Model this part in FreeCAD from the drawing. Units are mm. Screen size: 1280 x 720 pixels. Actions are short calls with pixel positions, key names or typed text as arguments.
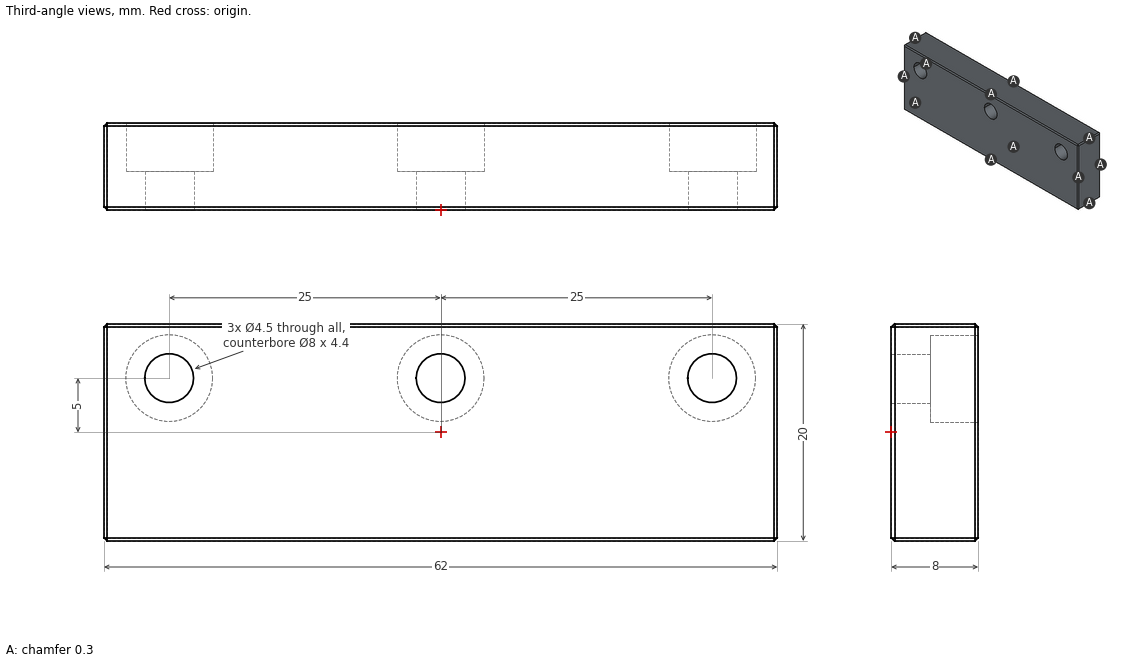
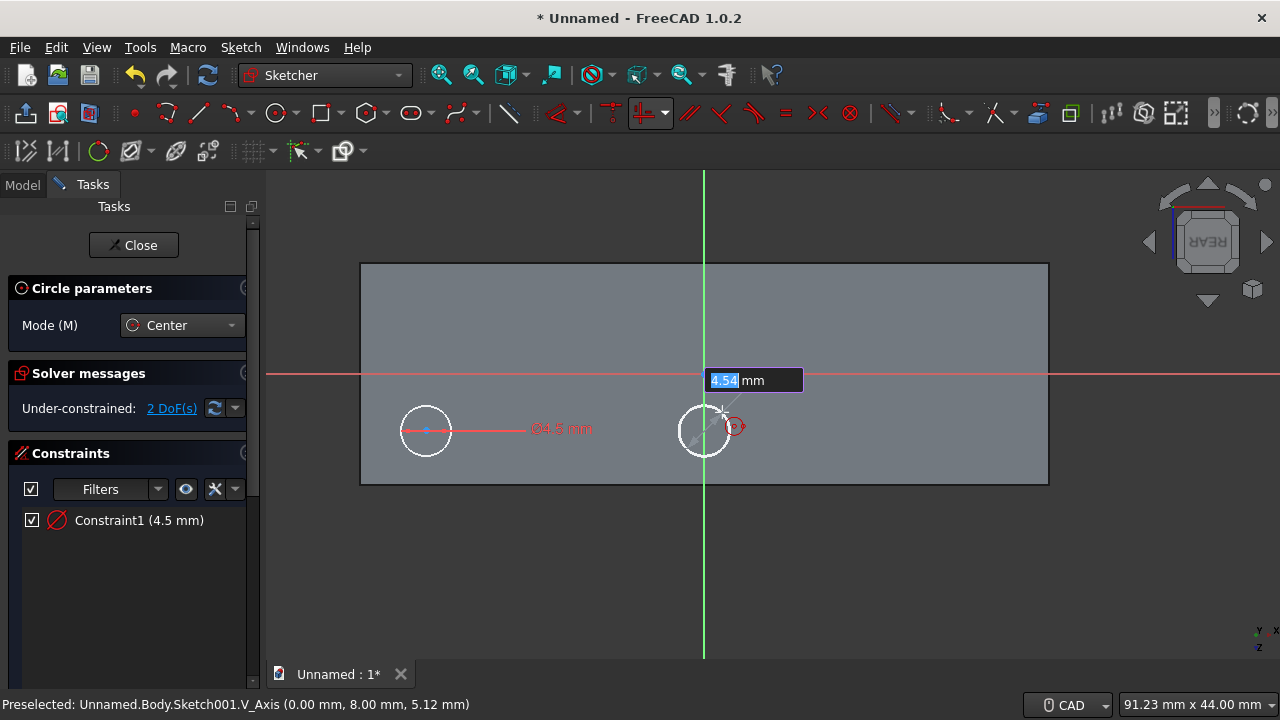
text(4.5)
key(Return)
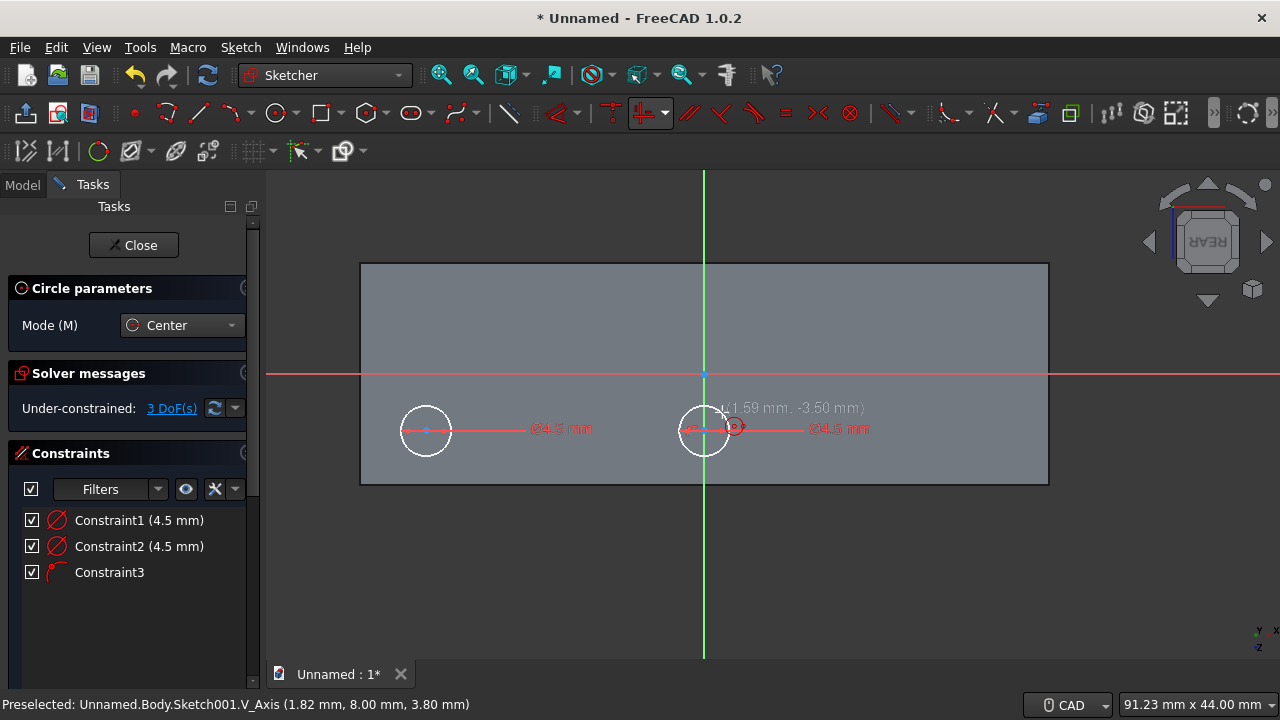
click(982, 430)
move(1000, 412)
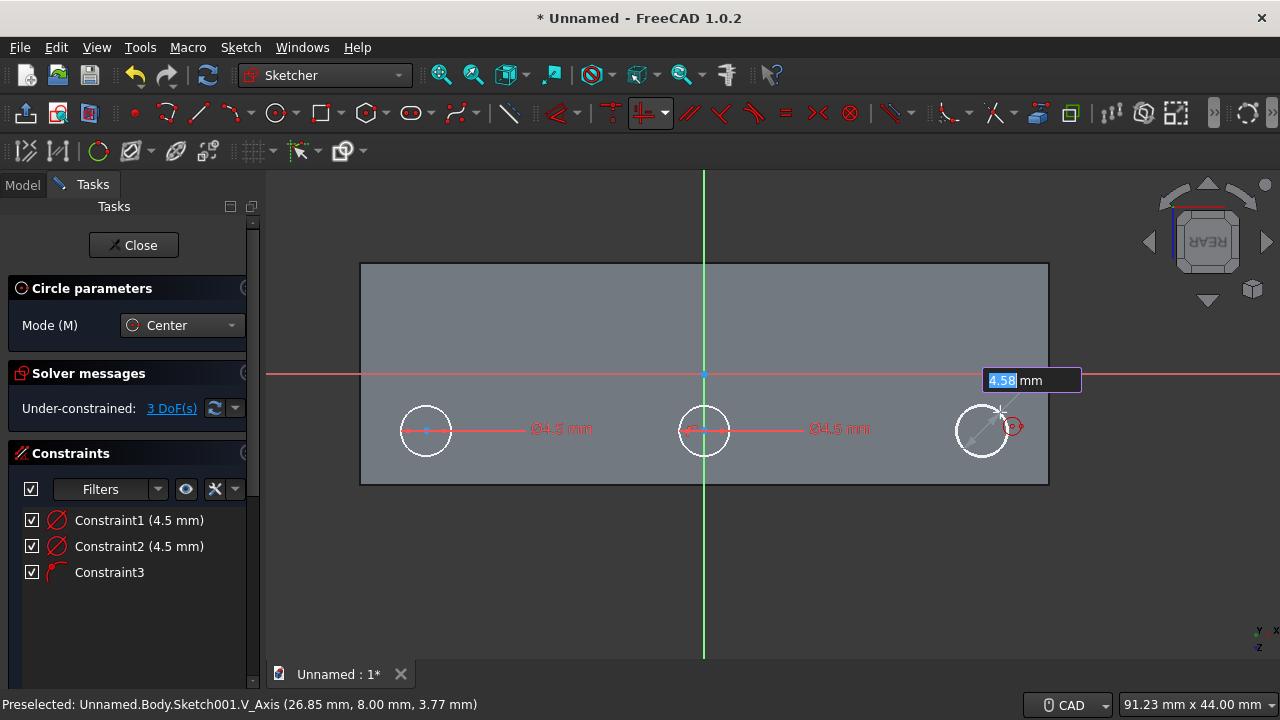
text(4.5)
key(Return)
key(Escape)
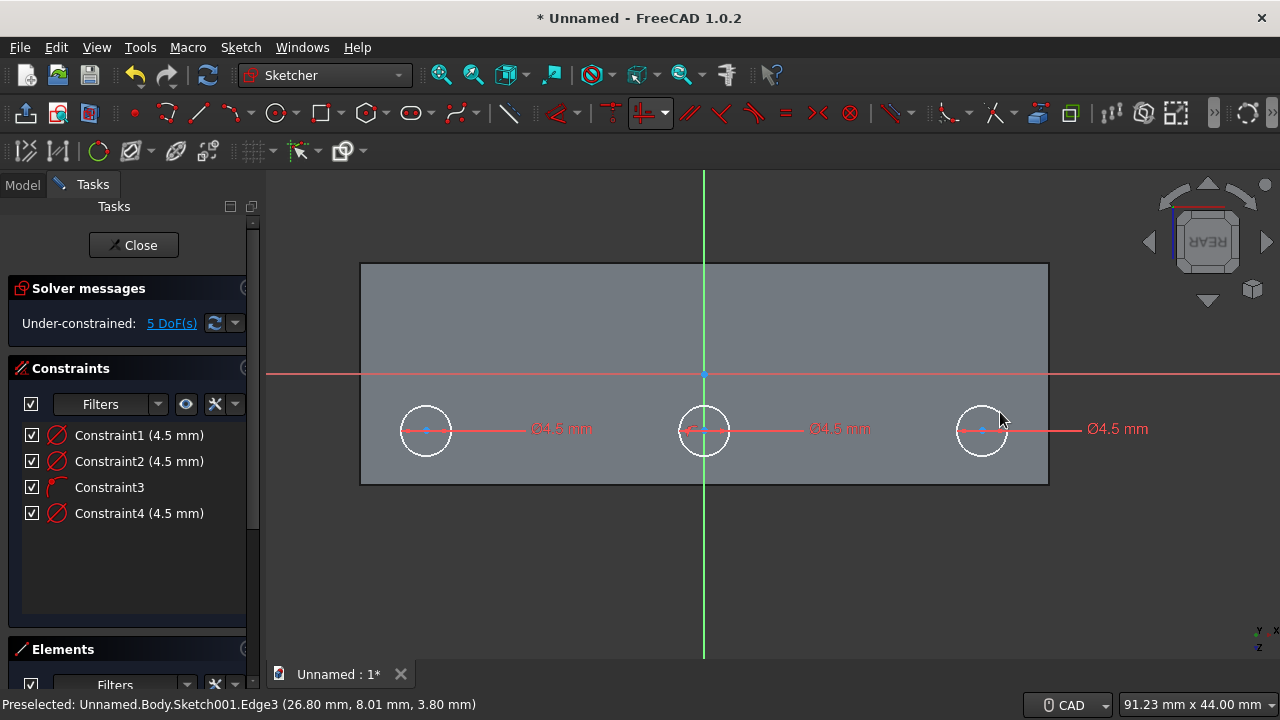
click(426, 431)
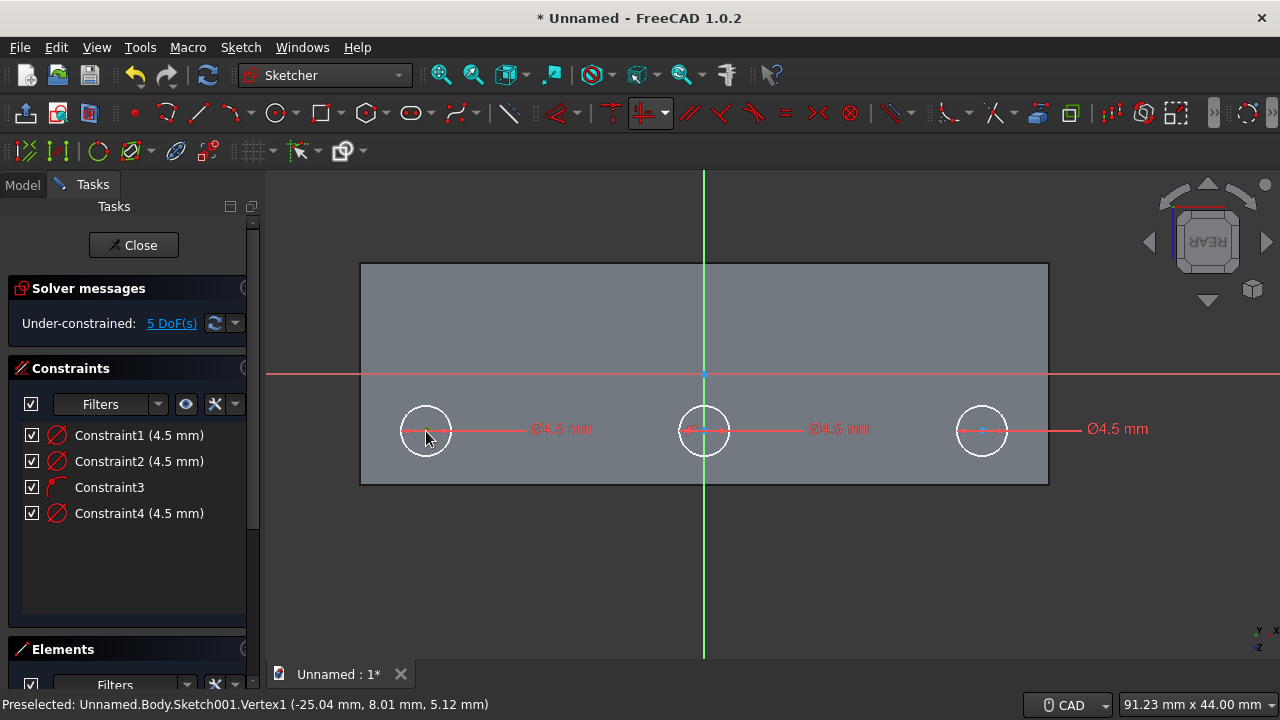
click(704, 431)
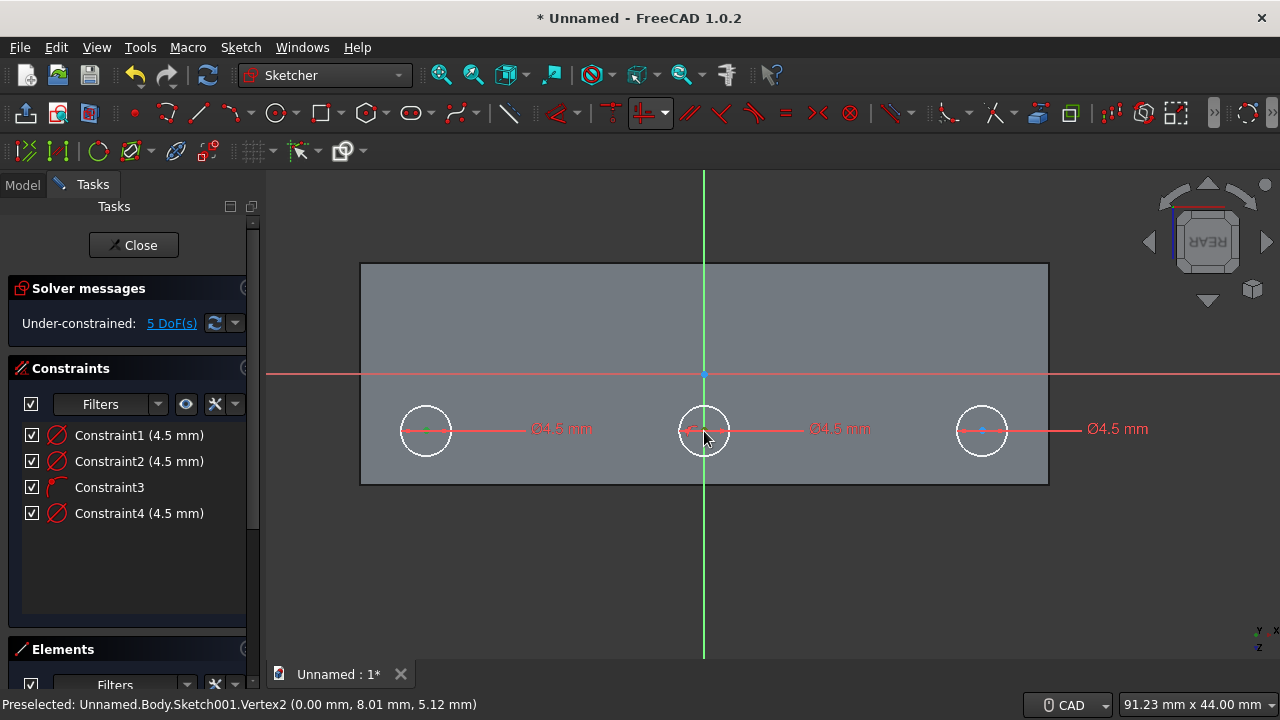
key(h)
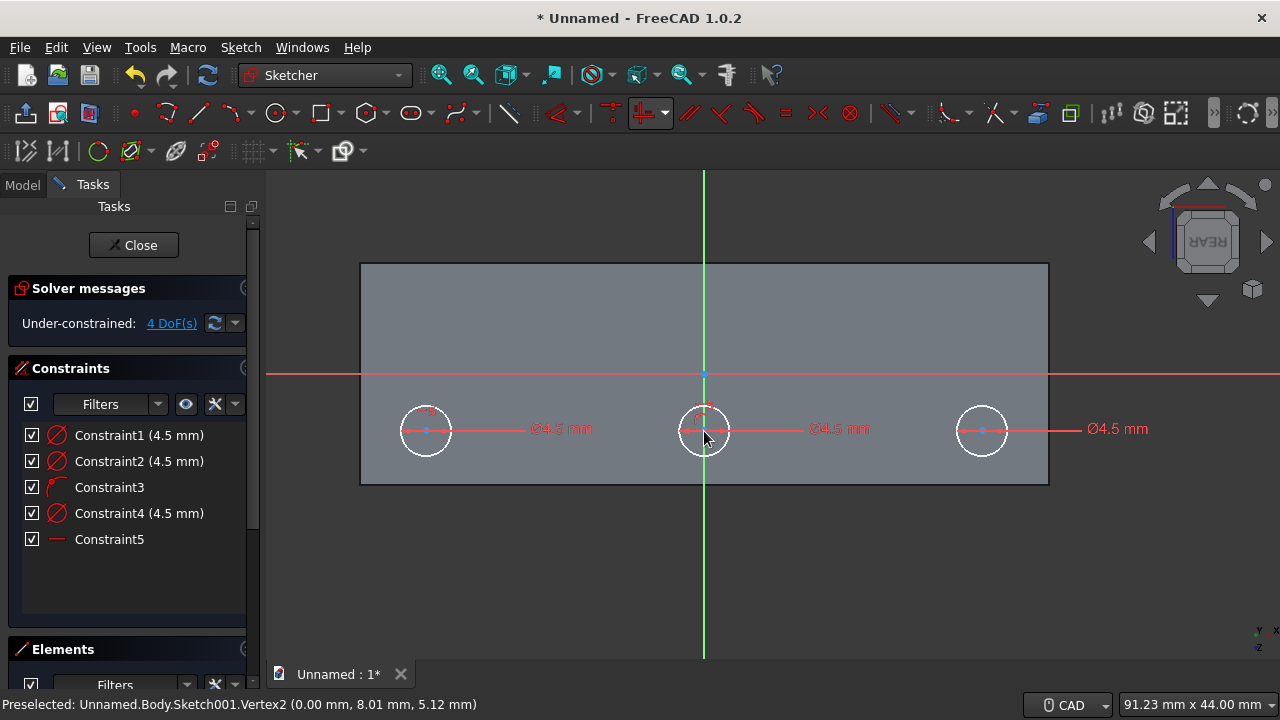
click(704, 431)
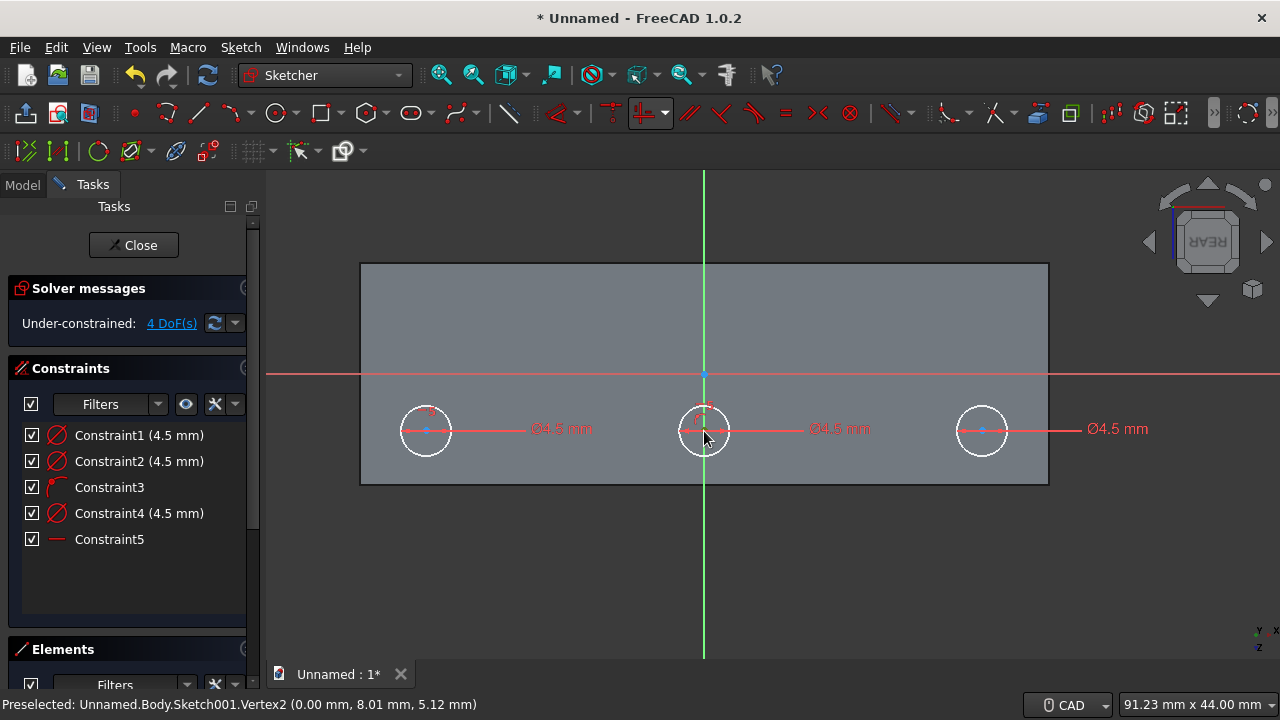
click(982, 431)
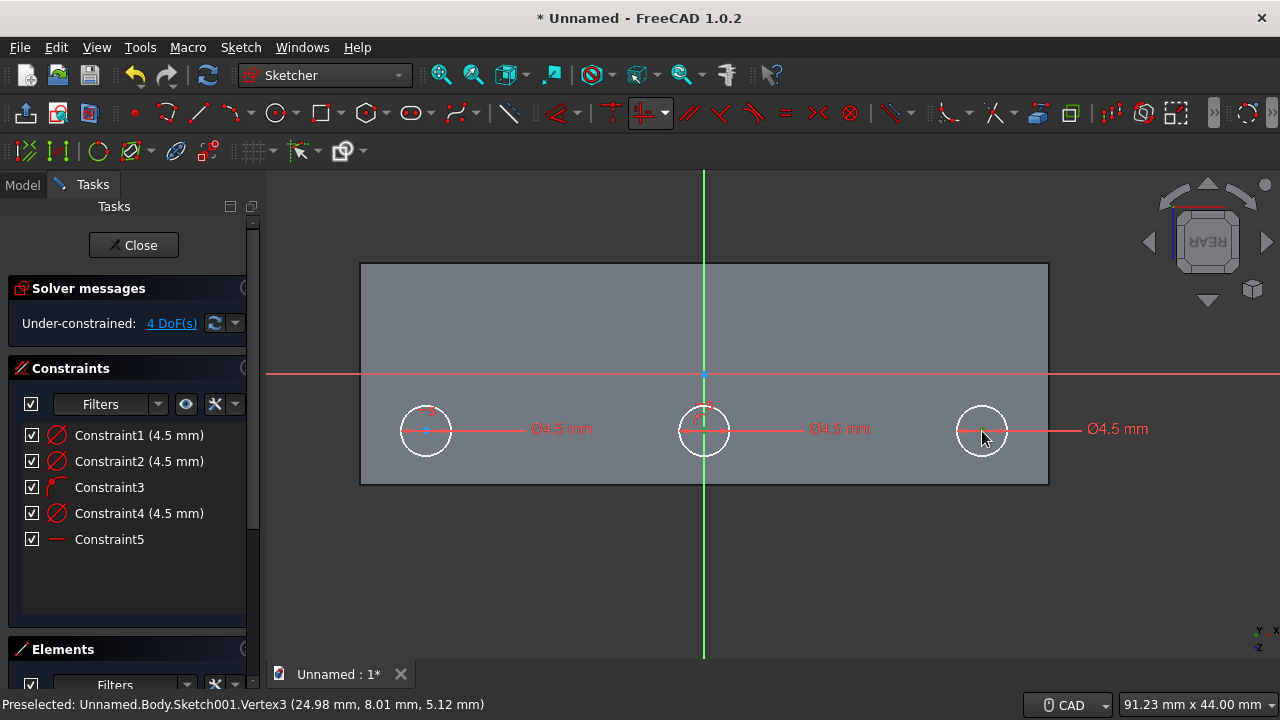
key(h)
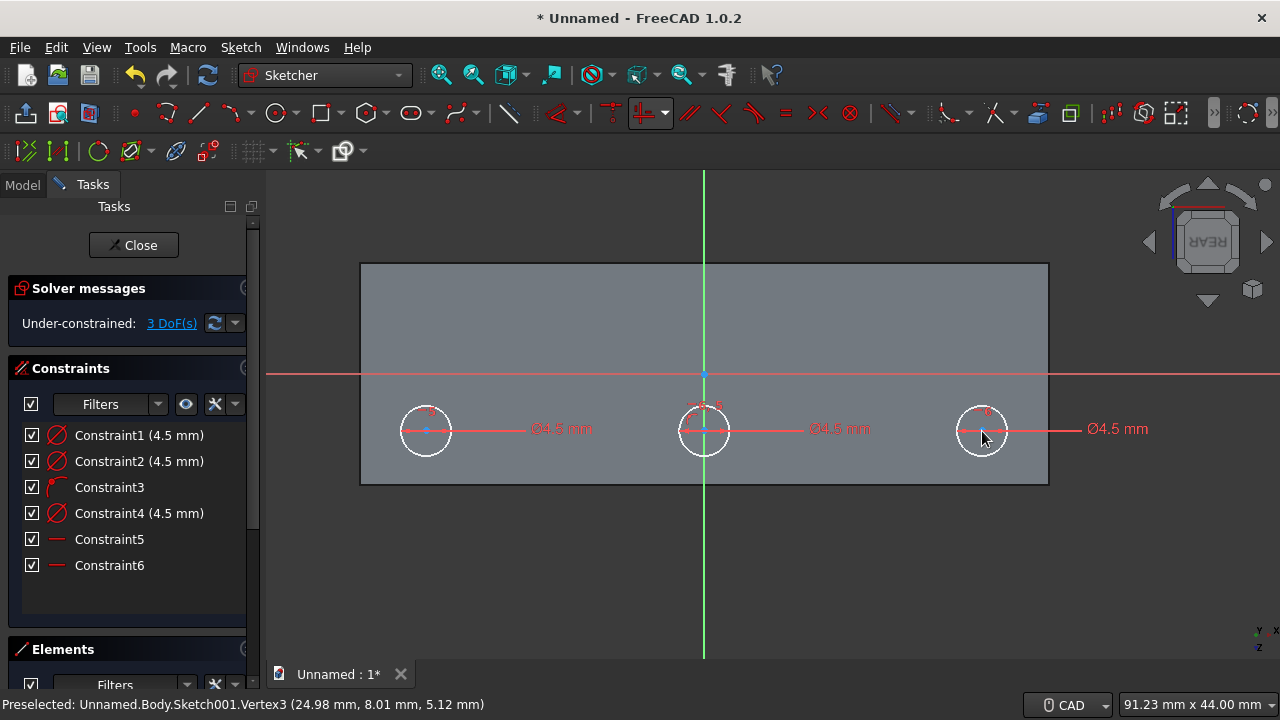
key(d)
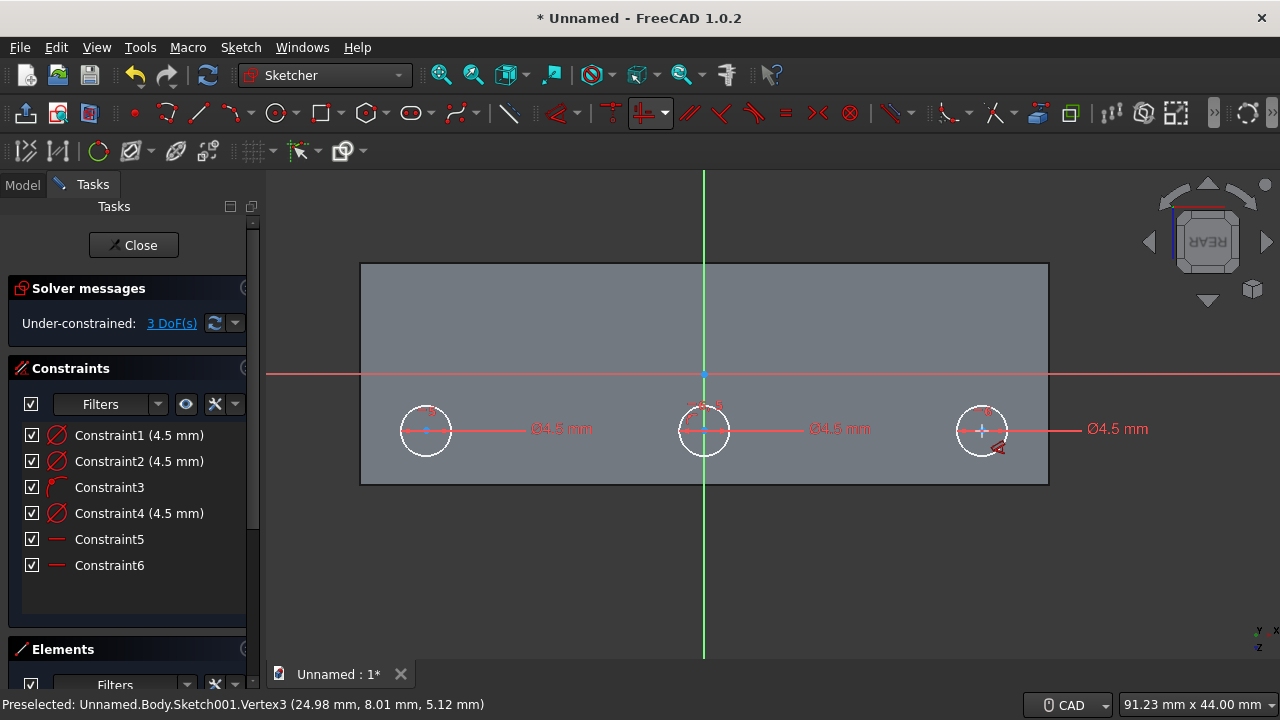
click(426, 431)
click(392, 403)